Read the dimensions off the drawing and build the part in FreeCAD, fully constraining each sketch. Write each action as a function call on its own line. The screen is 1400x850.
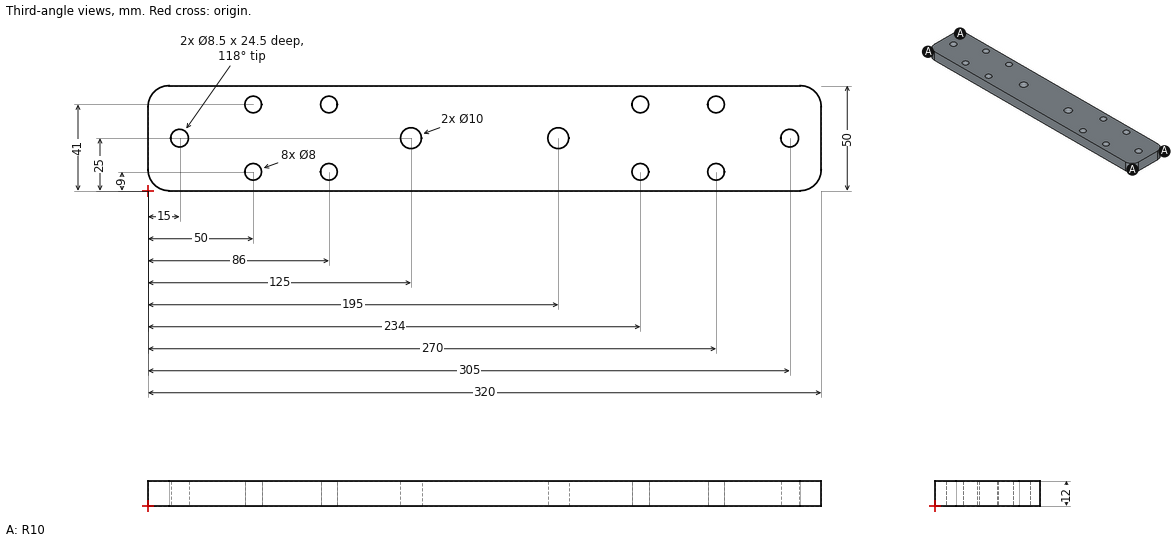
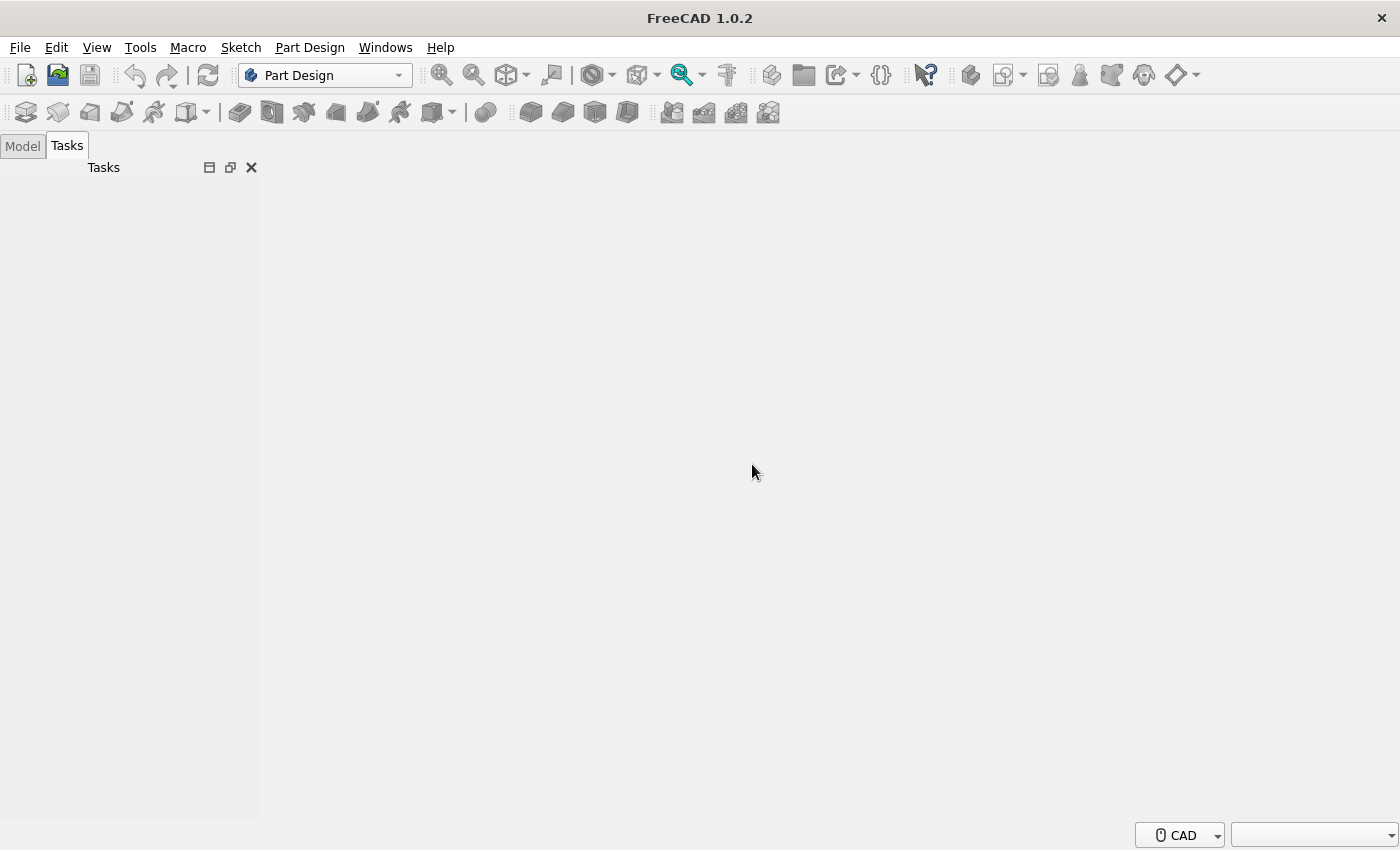
click(26, 76)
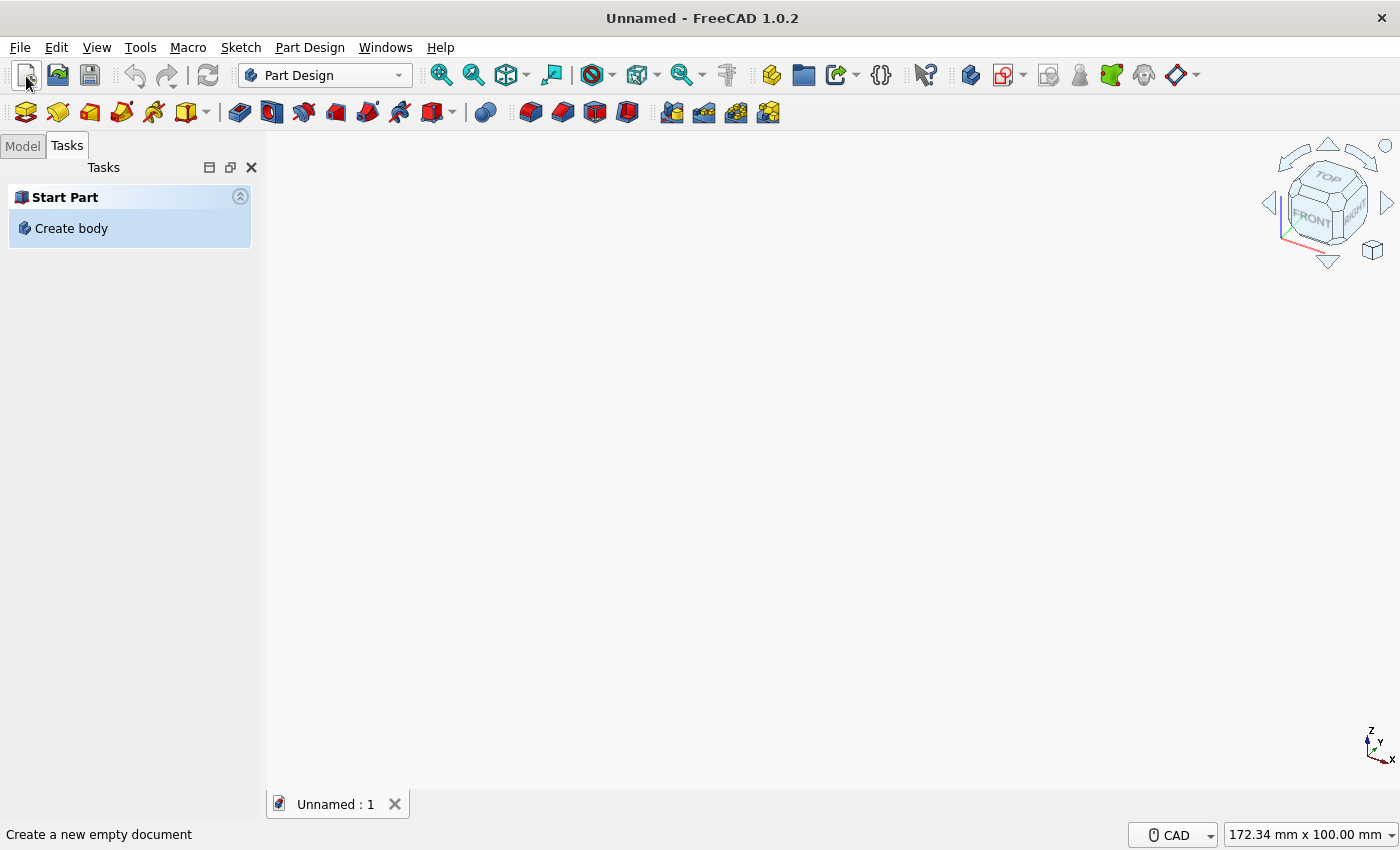
click(1004, 76)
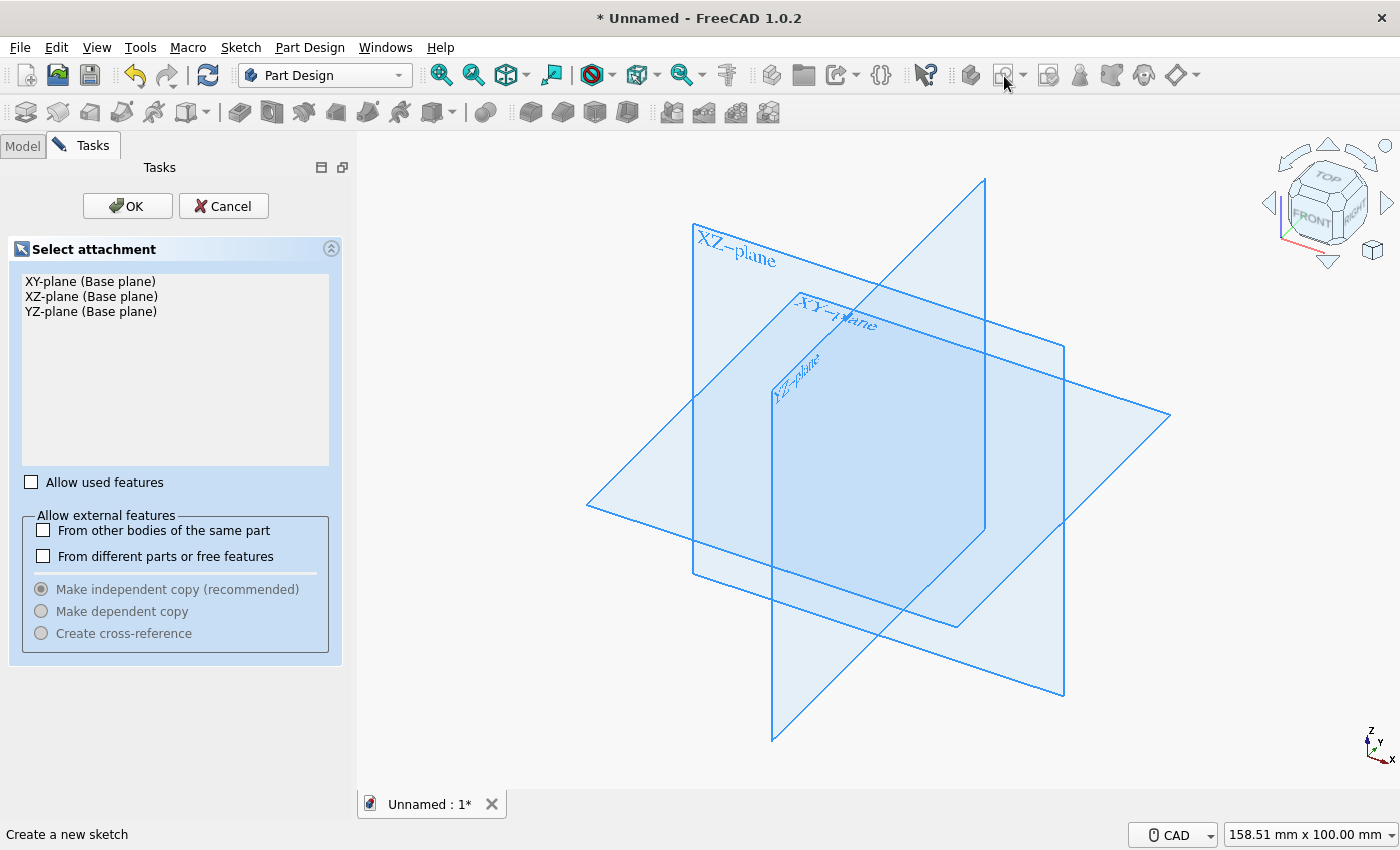
click(82, 282)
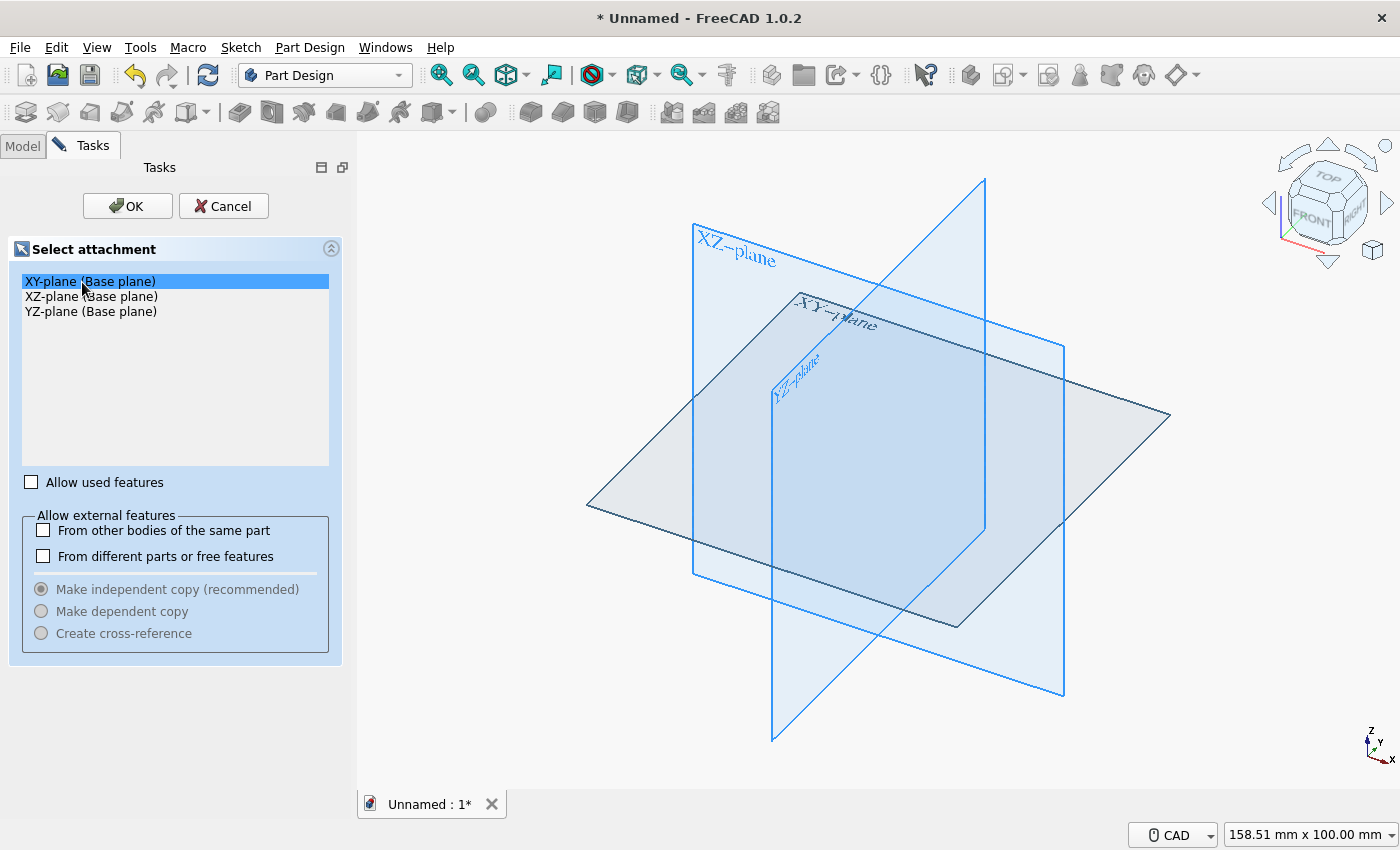
click(128, 206)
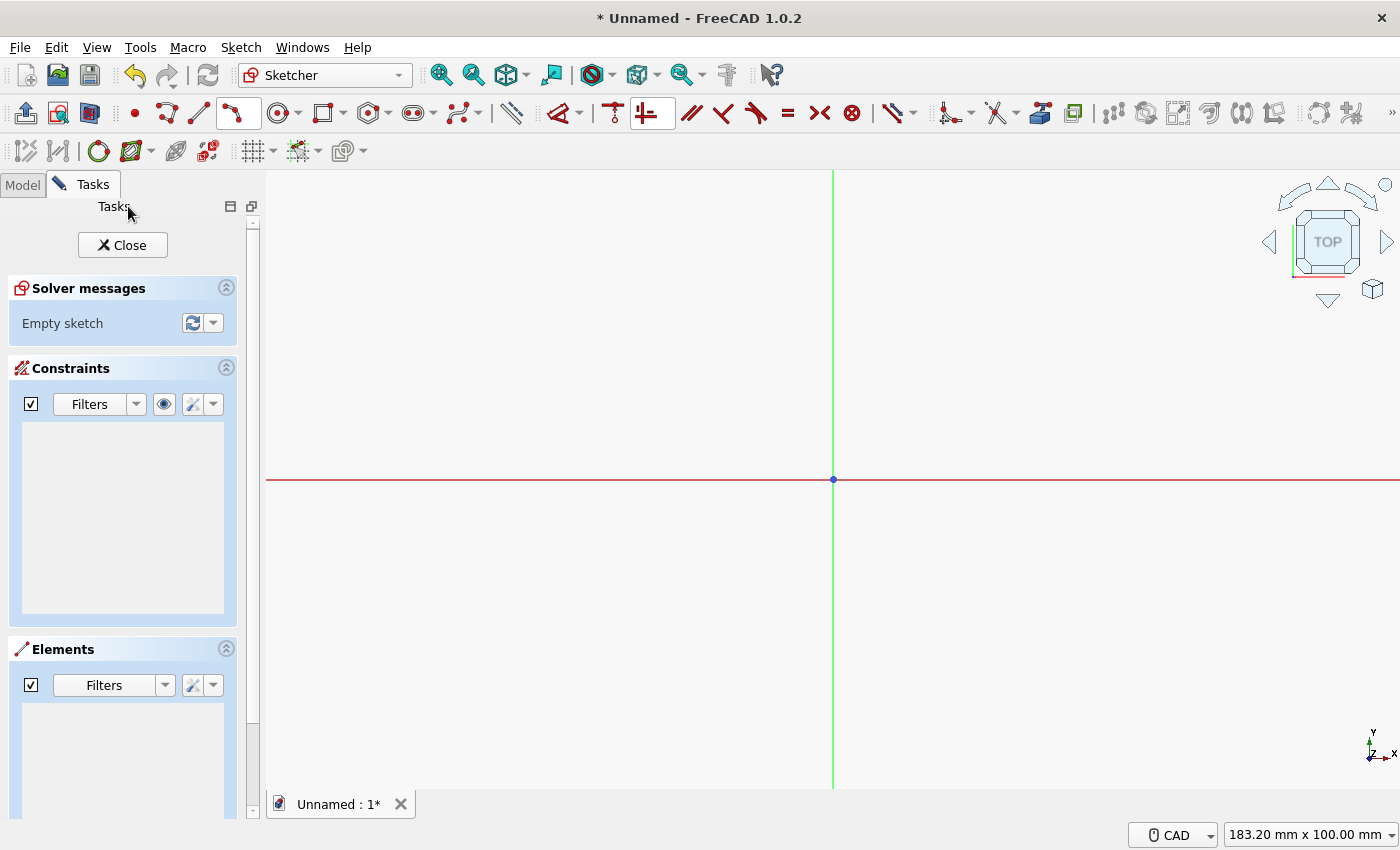
scroll(308, 546, down, 6)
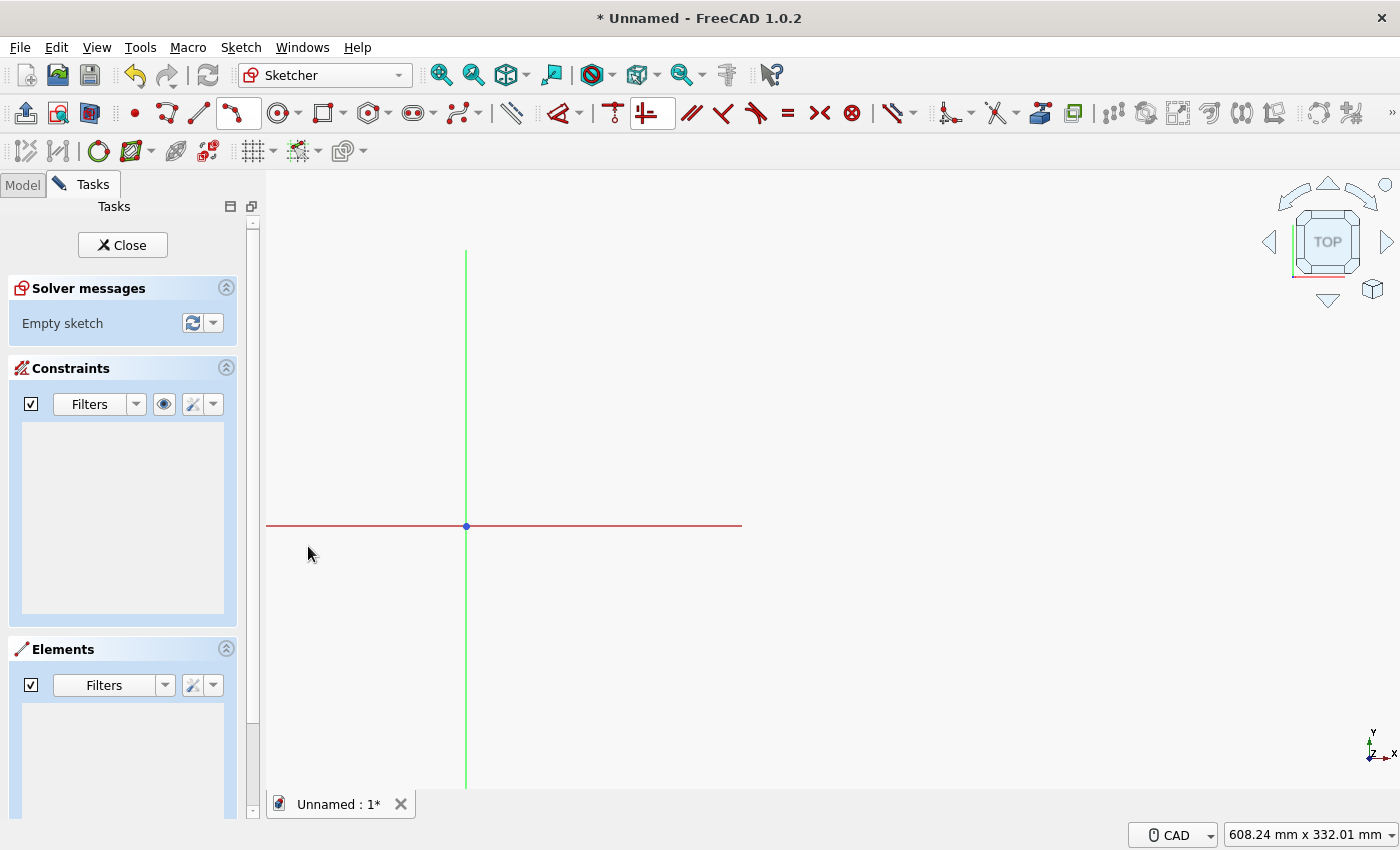
click(324, 114)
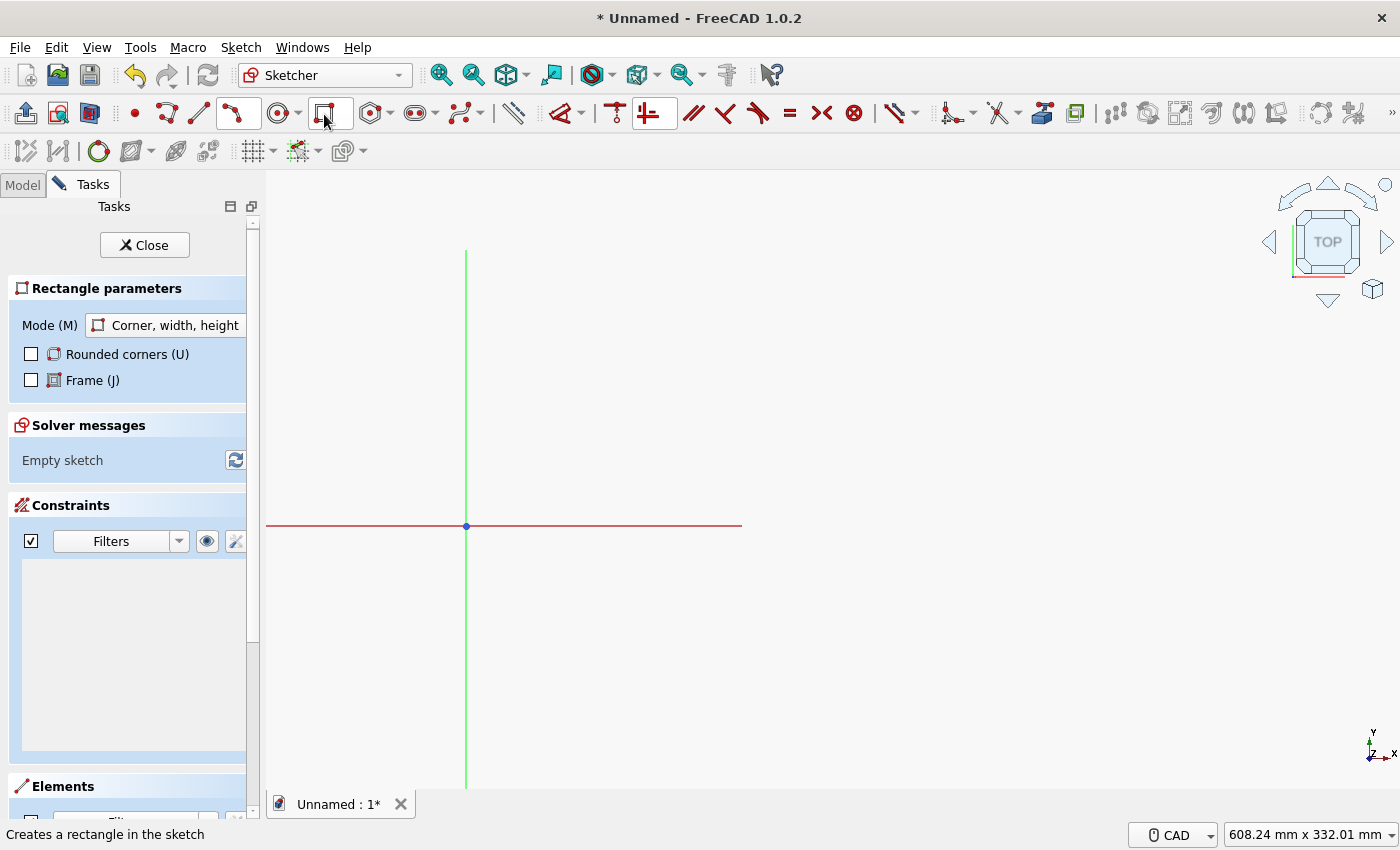
click(466, 526)
click(1063, 433)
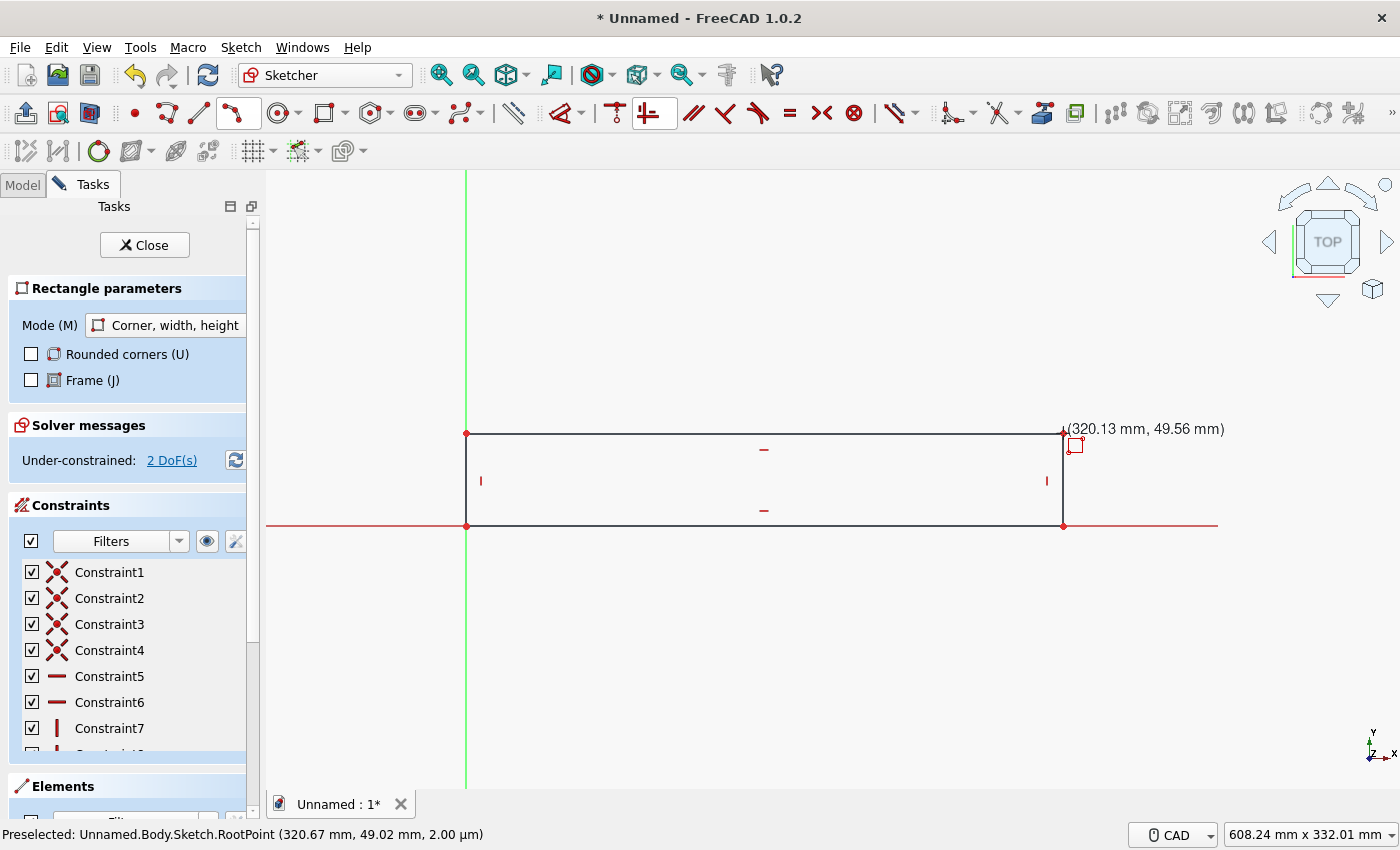
click(278, 114)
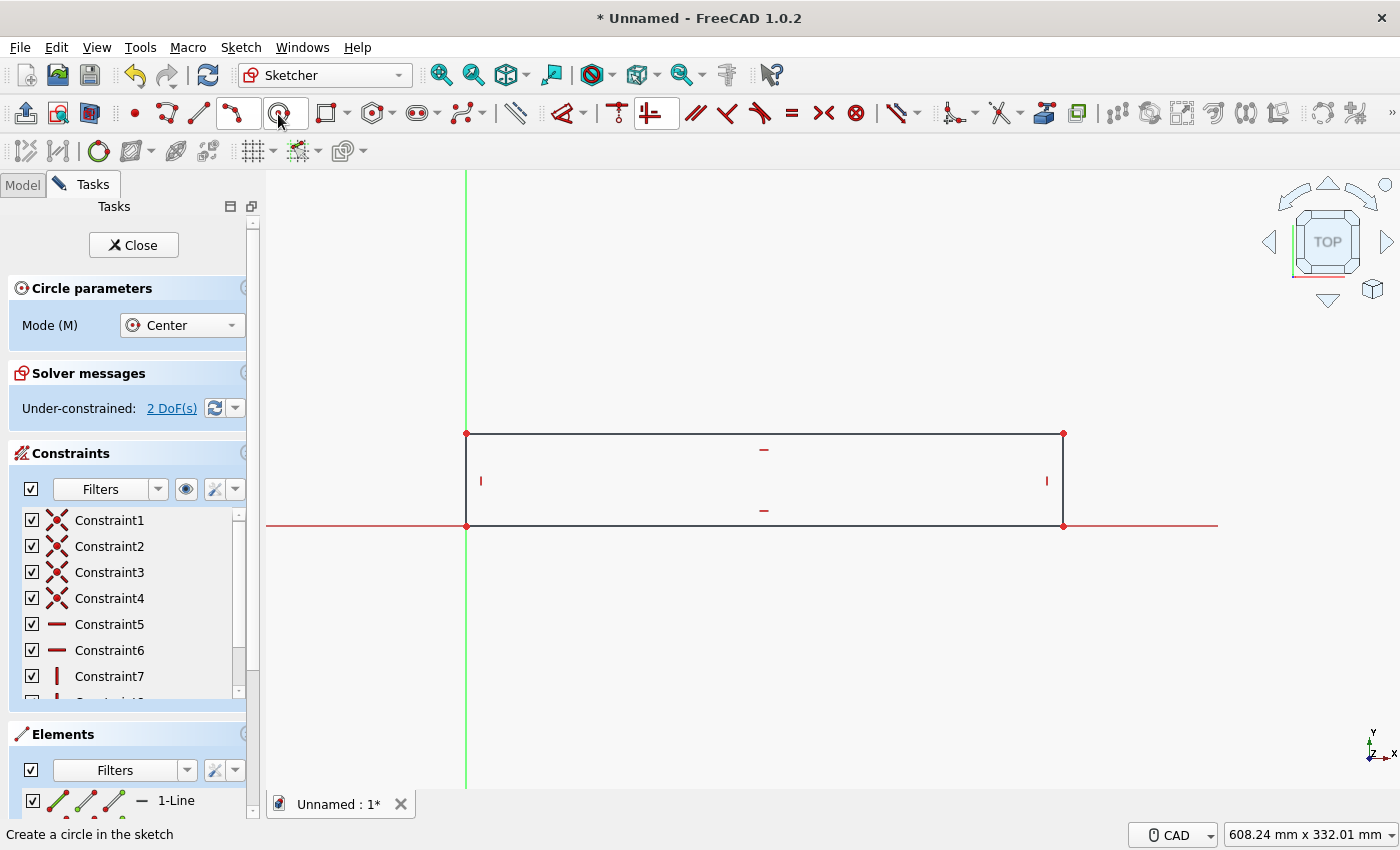
scroll(559, 510, up, 6)